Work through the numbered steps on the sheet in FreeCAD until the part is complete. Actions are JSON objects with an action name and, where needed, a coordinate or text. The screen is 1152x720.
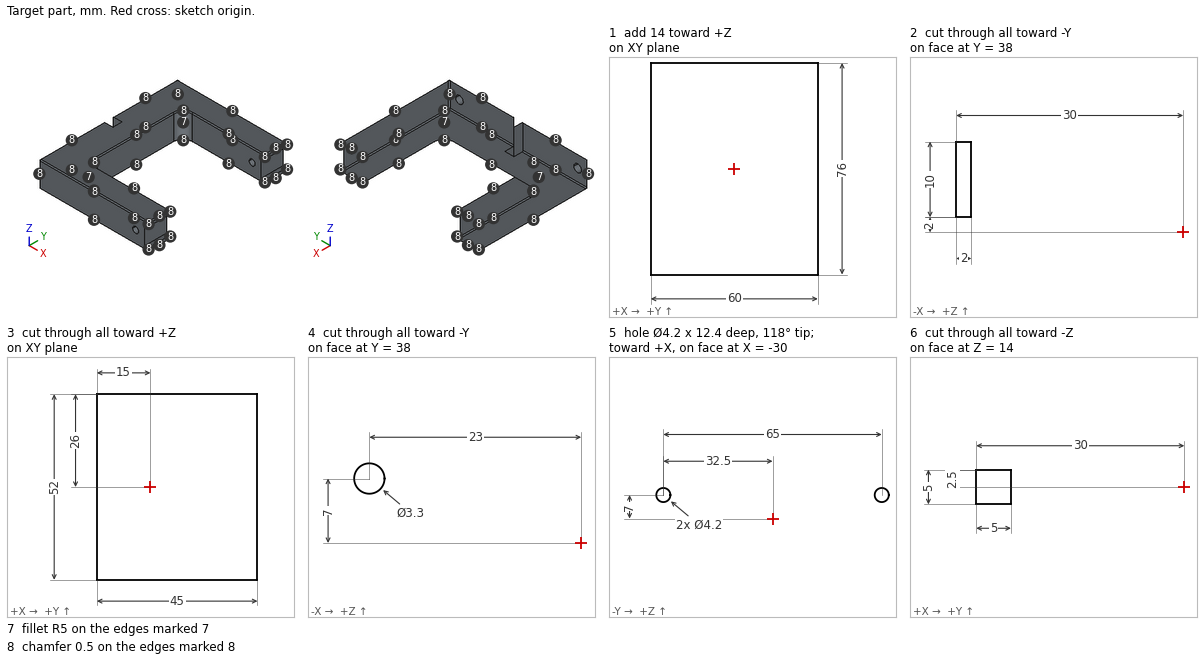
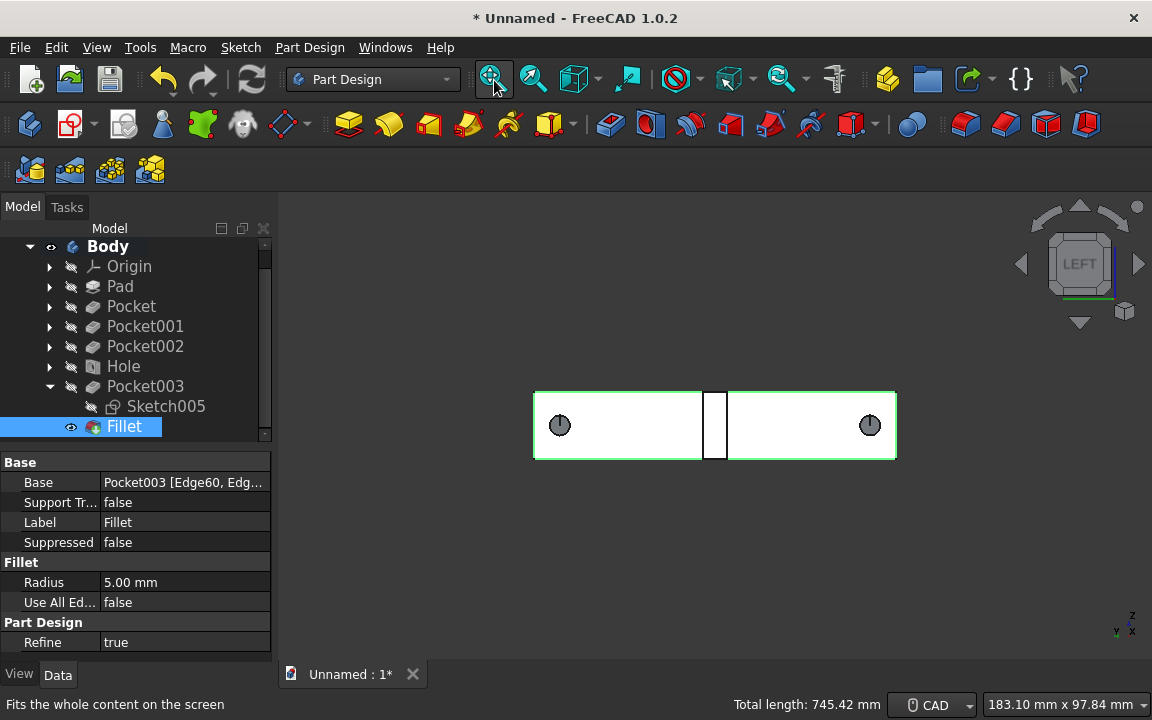
{"action": "key", "text": "v 3"}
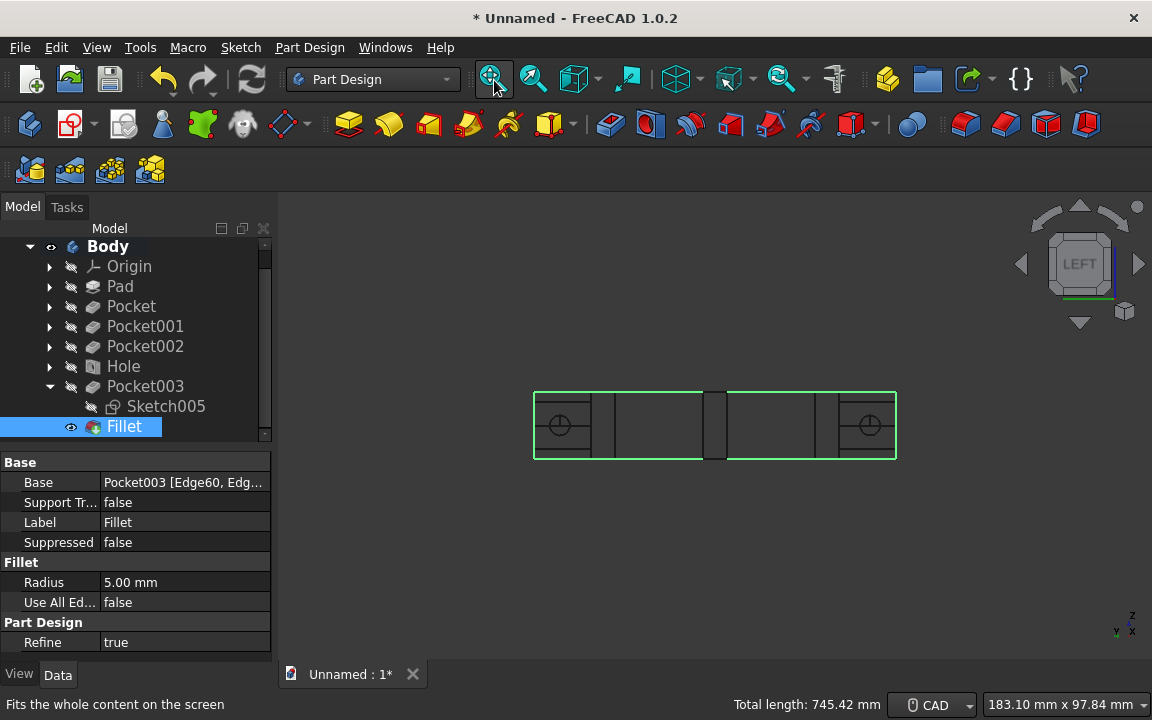
{"action": "key", "text": "0"}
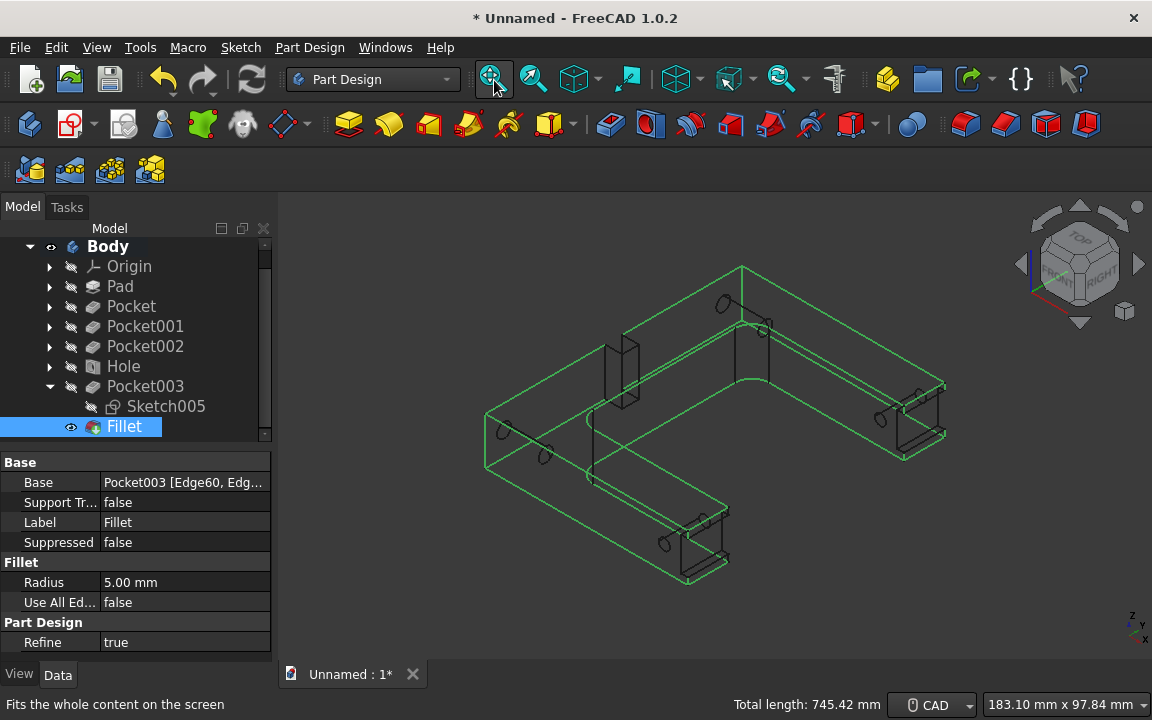
{"action": "scroll", "coordinate": [729, 510], "scroll_direction": "up", "scroll_amount": 8}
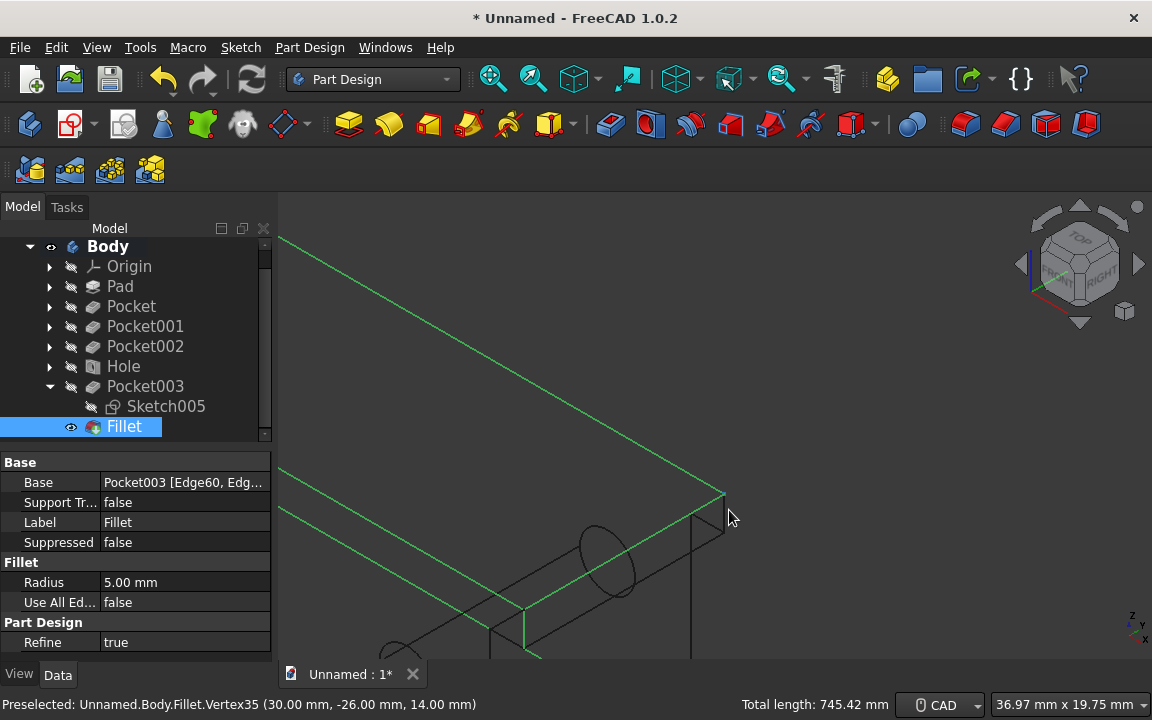
{"action": "left_click", "coordinate": [724, 512], "text": "ctrl"}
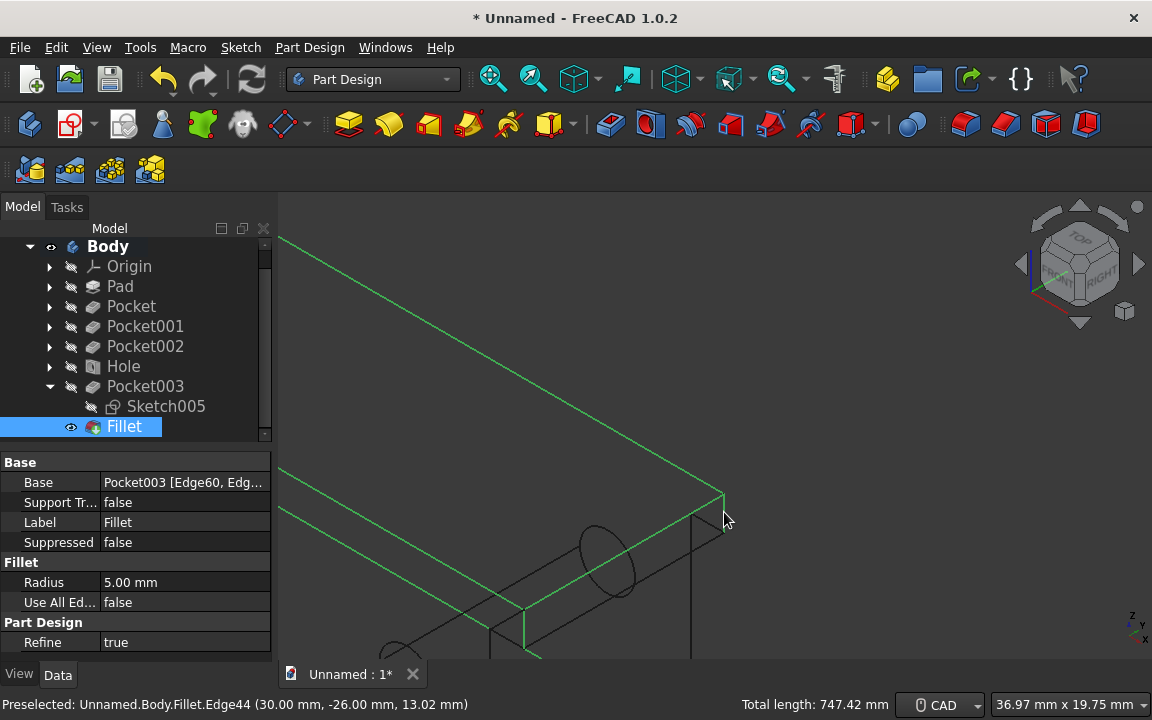
{"action": "key", "text": "v f"}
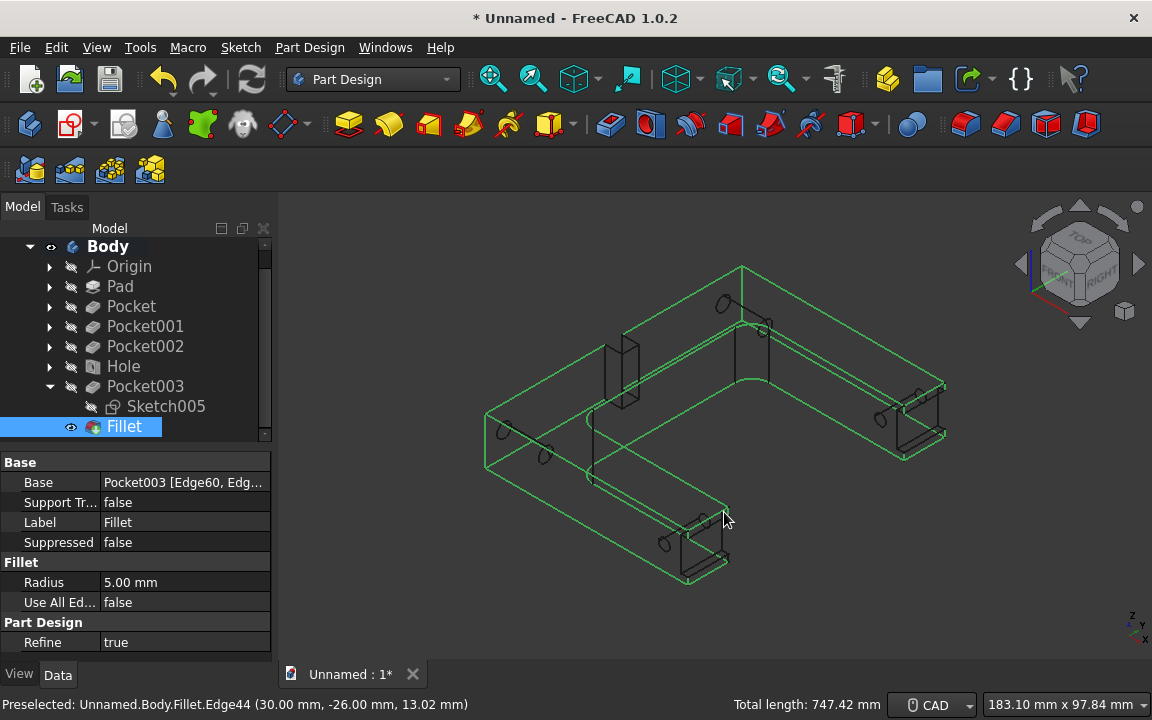
{"action": "key", "text": "2"}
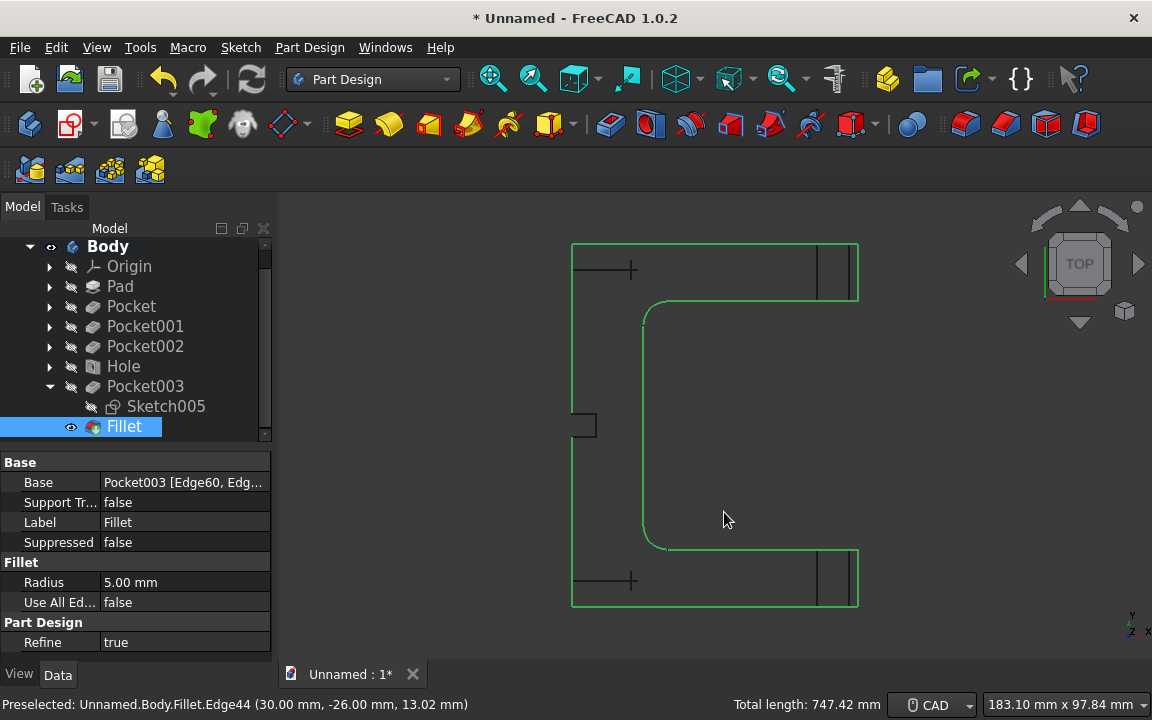
{"action": "scroll", "coordinate": [858, 549], "scroll_direction": "up", "scroll_amount": 8}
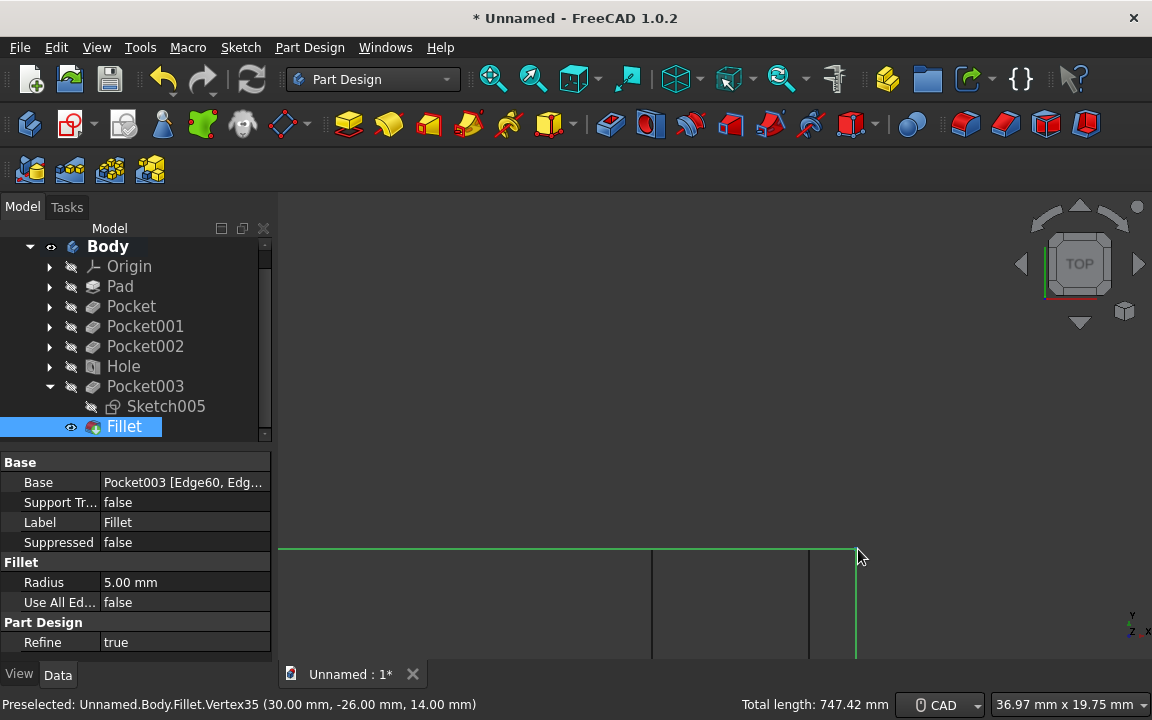
{"action": "key", "text": "v f"}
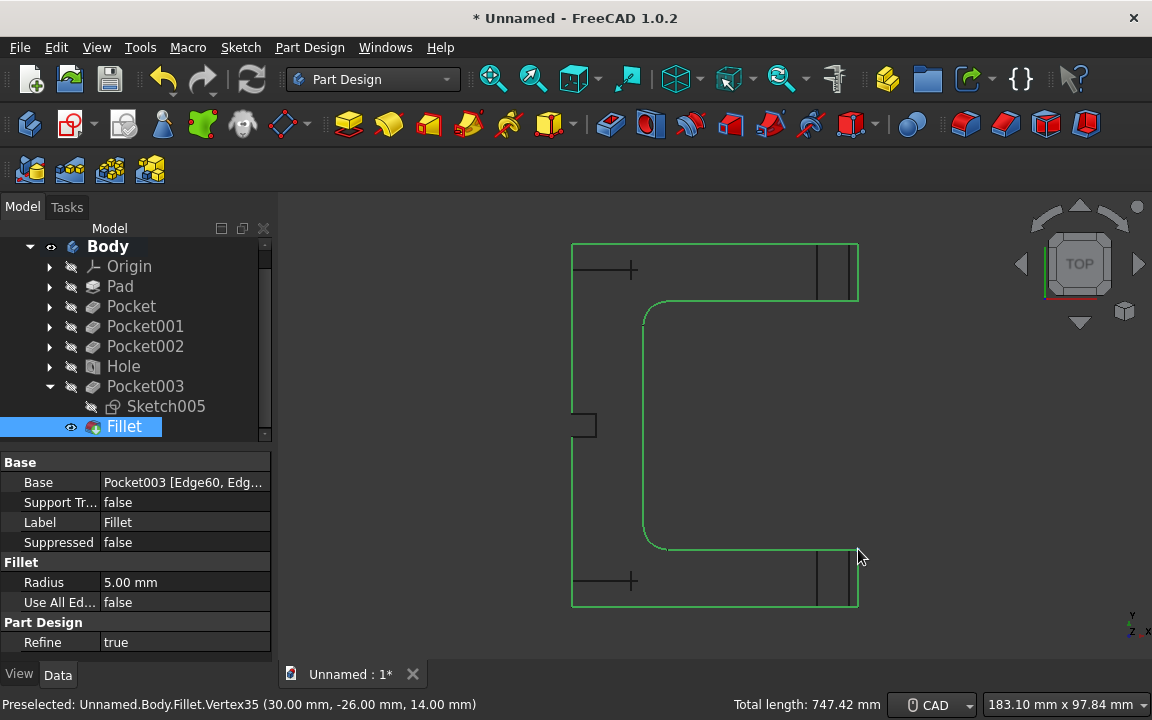
{"action": "key", "text": "1"}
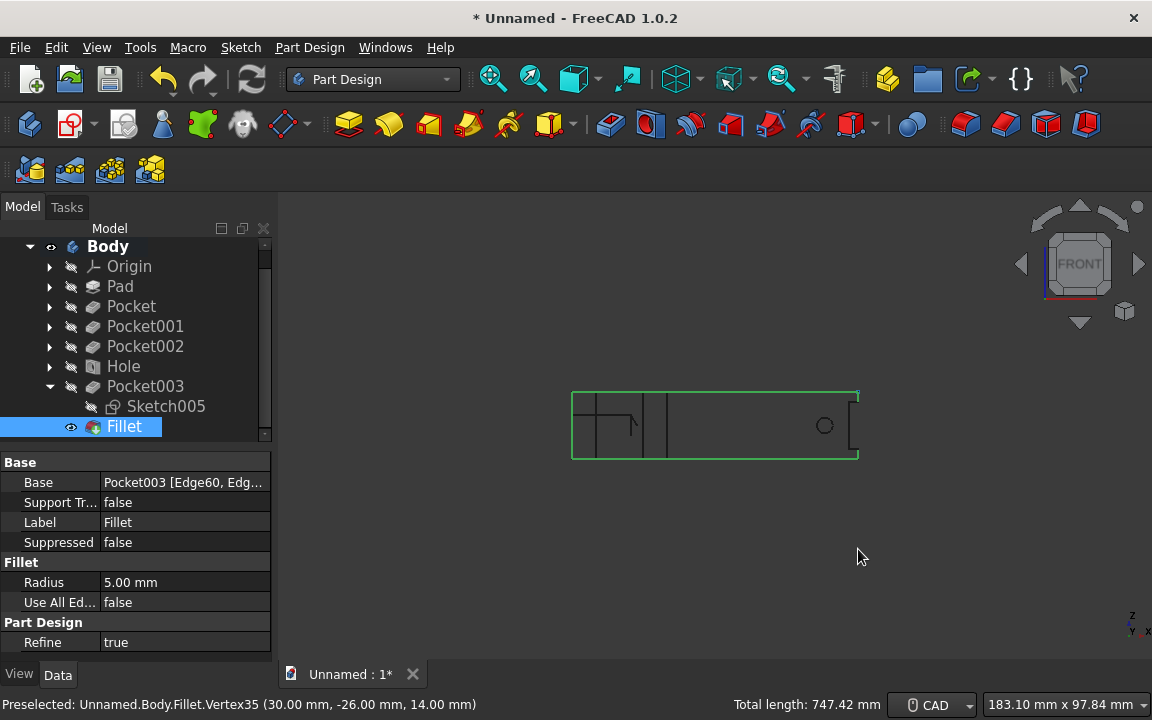
{"action": "key", "text": "v f"}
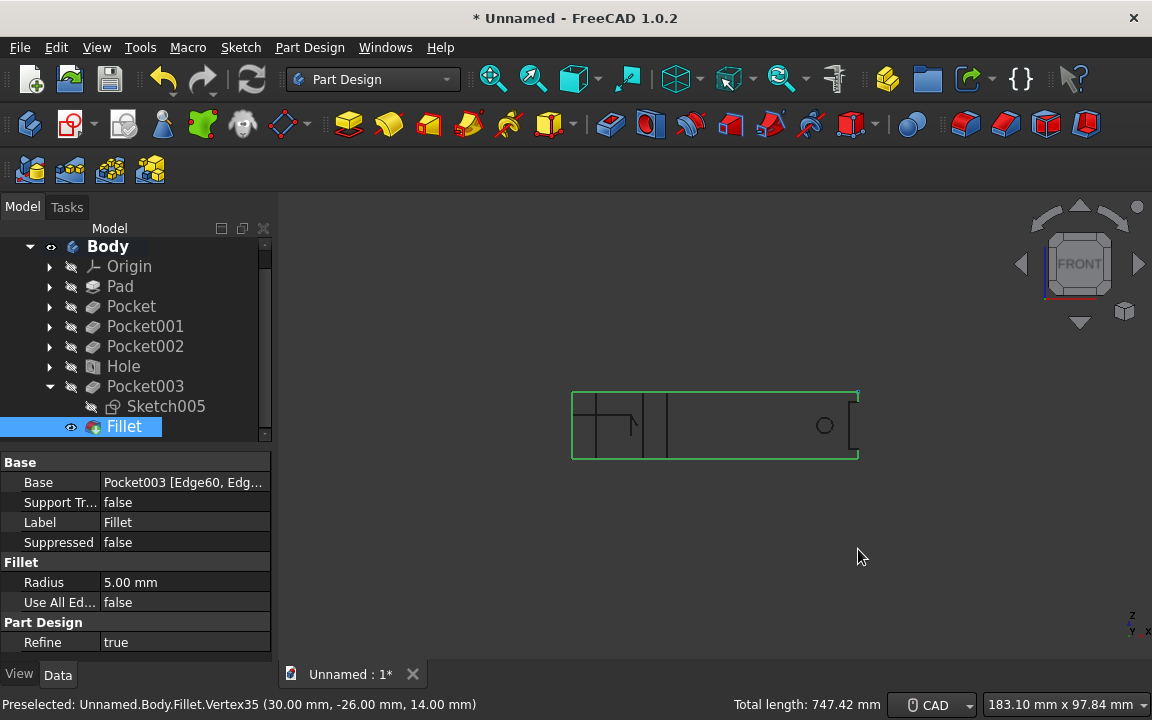
{"action": "scroll", "coordinate": [858, 453], "scroll_direction": "up", "scroll_amount": 8}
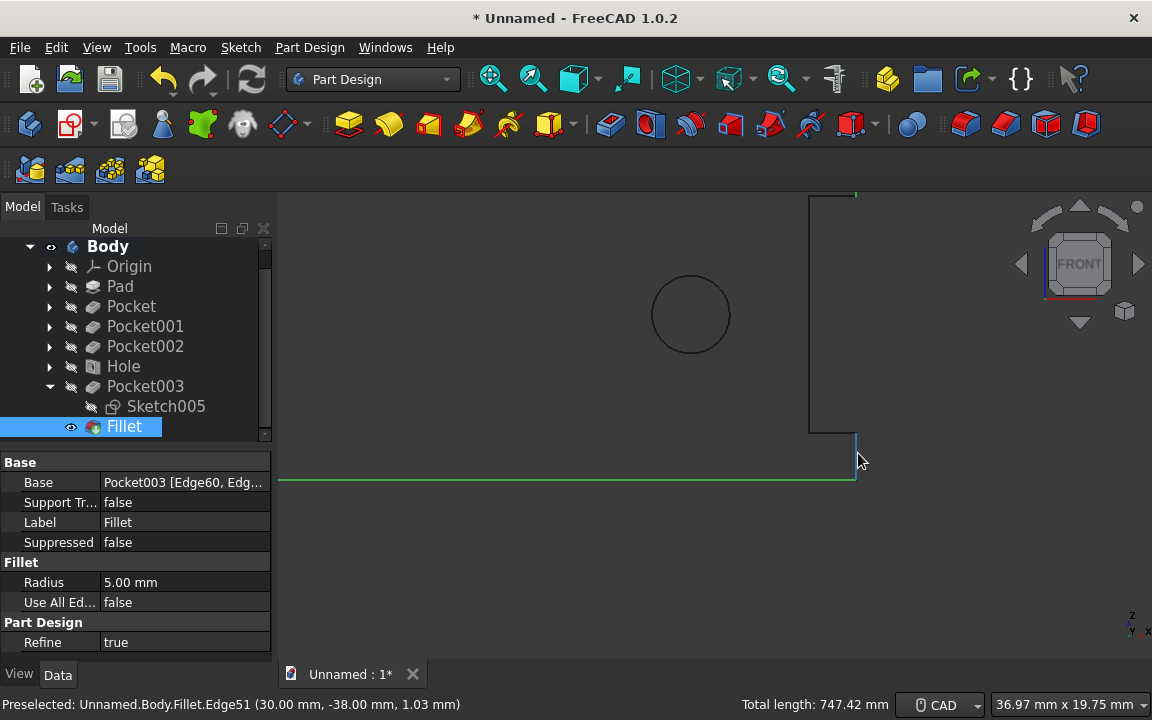
{"action": "left_click", "coordinate": [494, 80]}